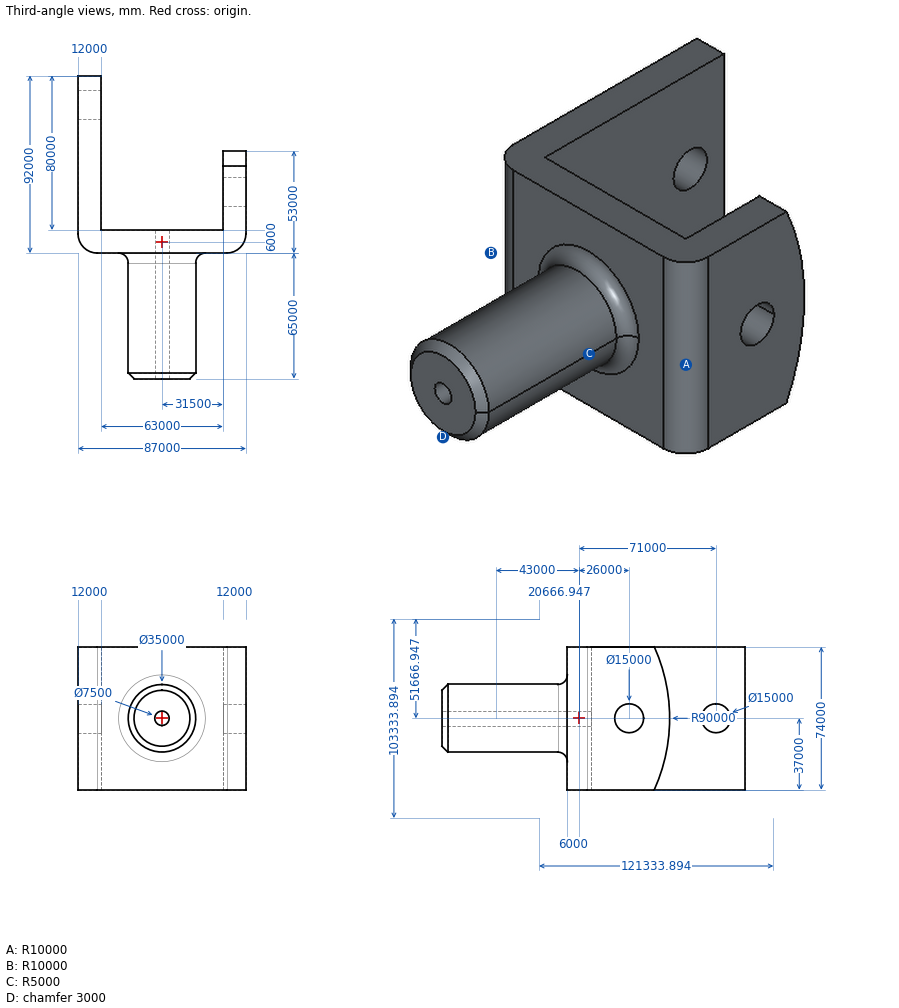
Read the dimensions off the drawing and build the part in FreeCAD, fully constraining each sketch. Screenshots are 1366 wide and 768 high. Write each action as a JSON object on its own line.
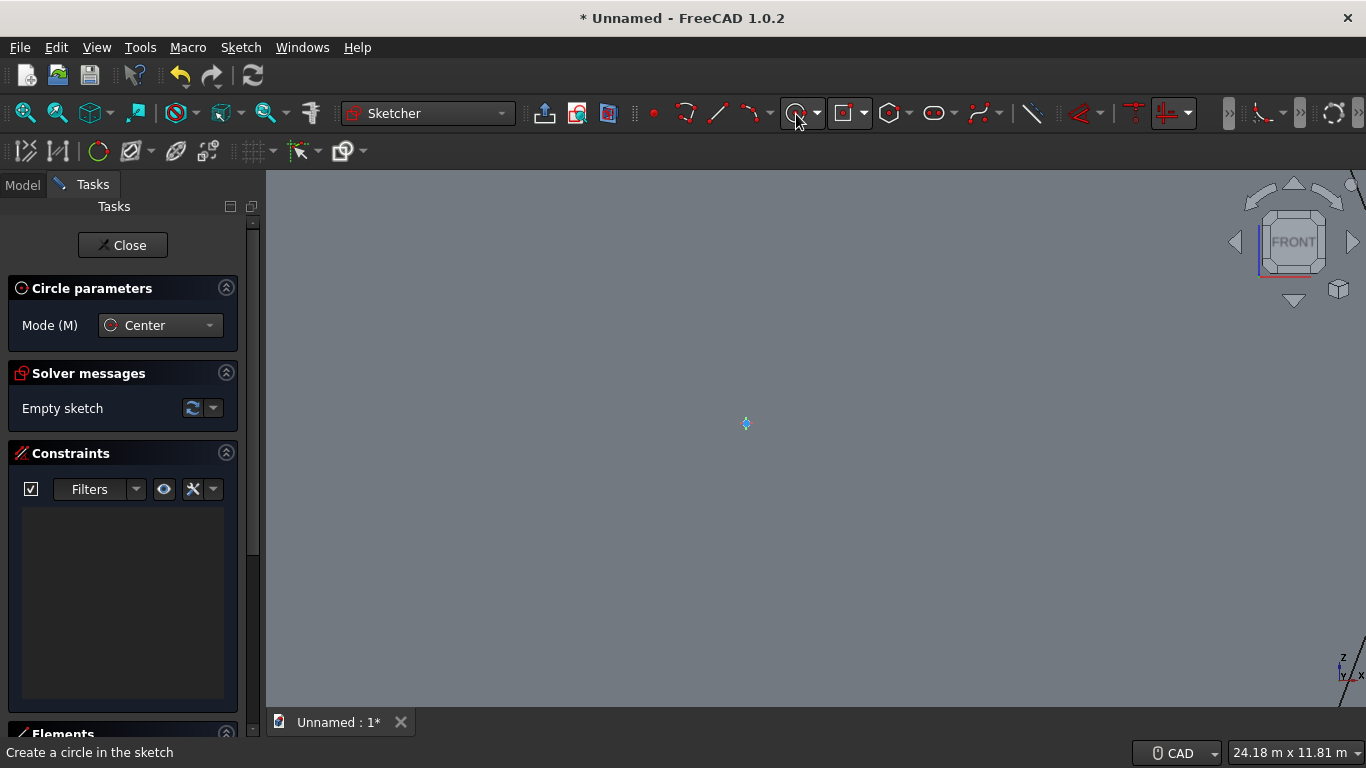
{"action": "left_click", "coordinate": [746, 423]}
{"action": "mouse_move", "coordinate": [867, 302]}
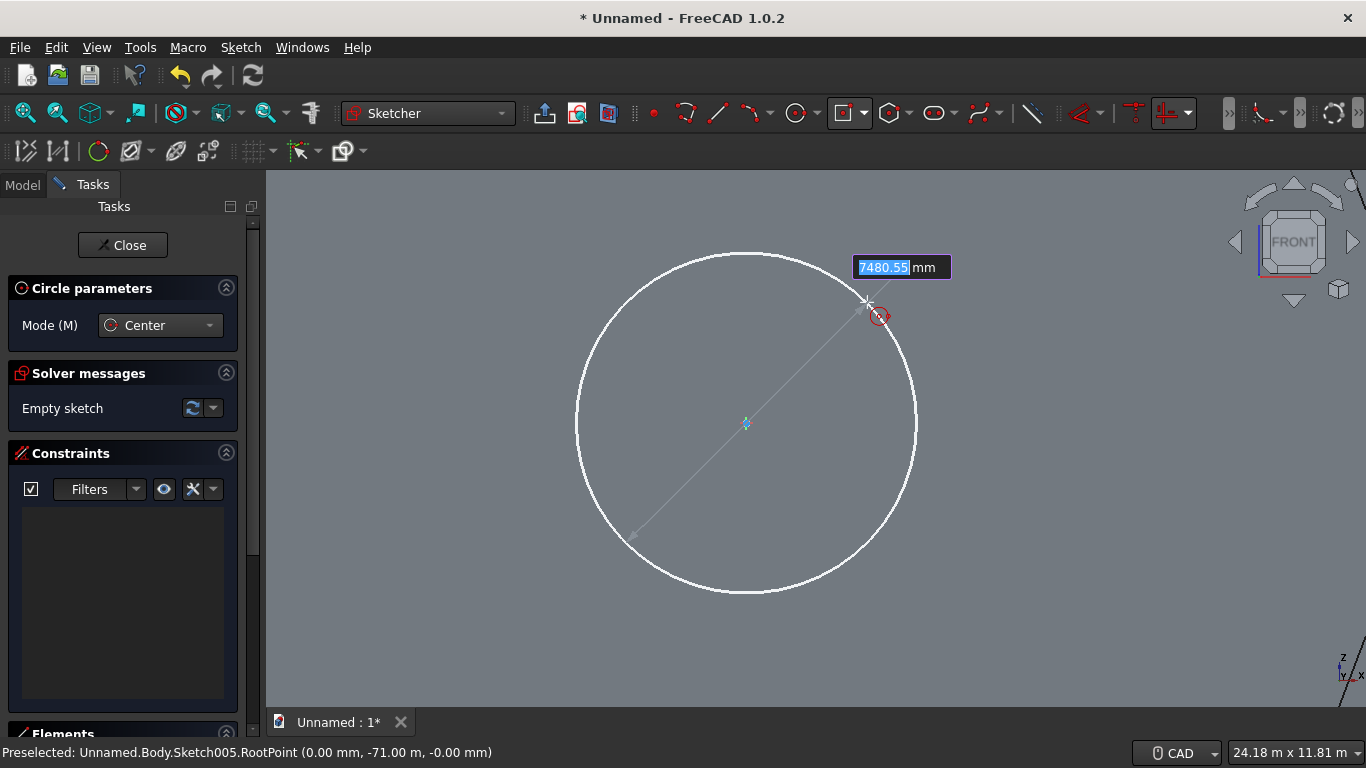
{"action": "type", "text": "7500"}
{"action": "key", "text": "Return"}
{"action": "key", "text": "Escape"}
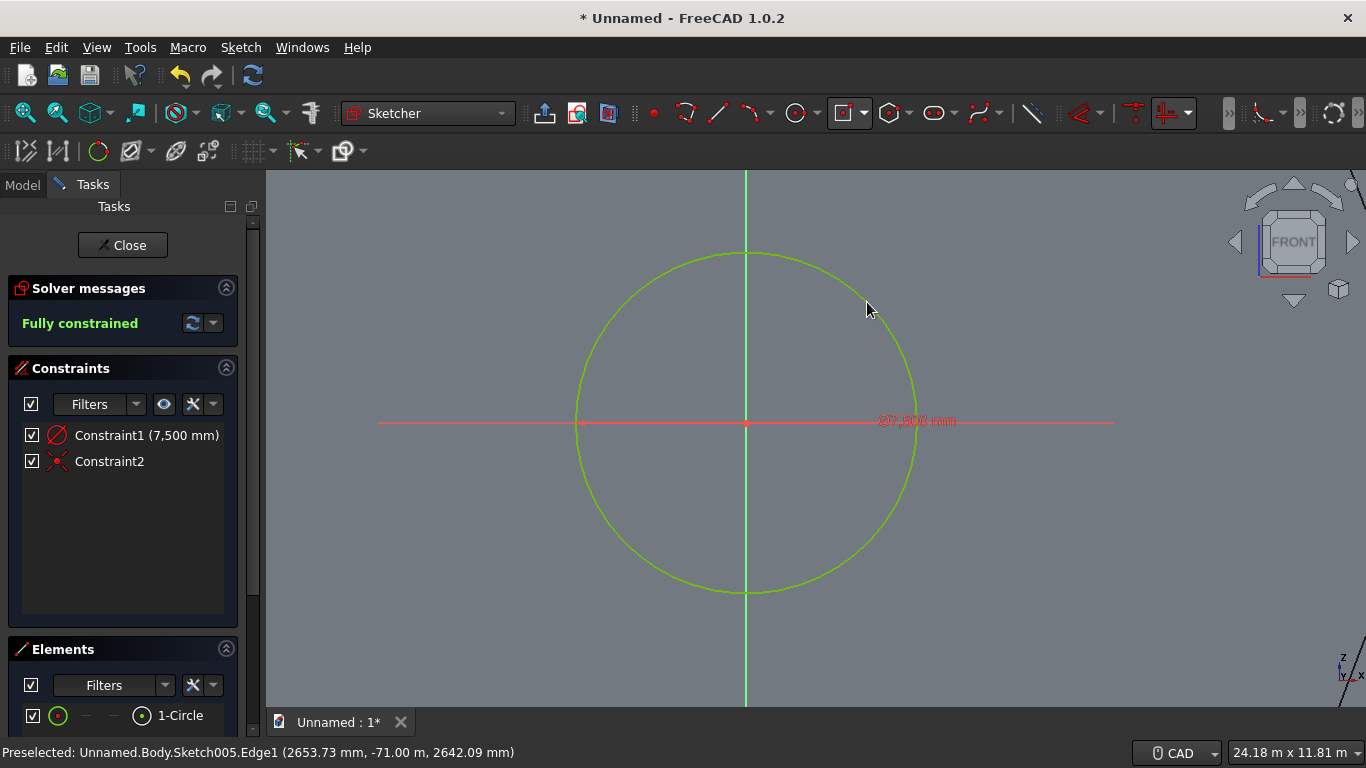
{"action": "left_click", "coordinate": [123, 245]}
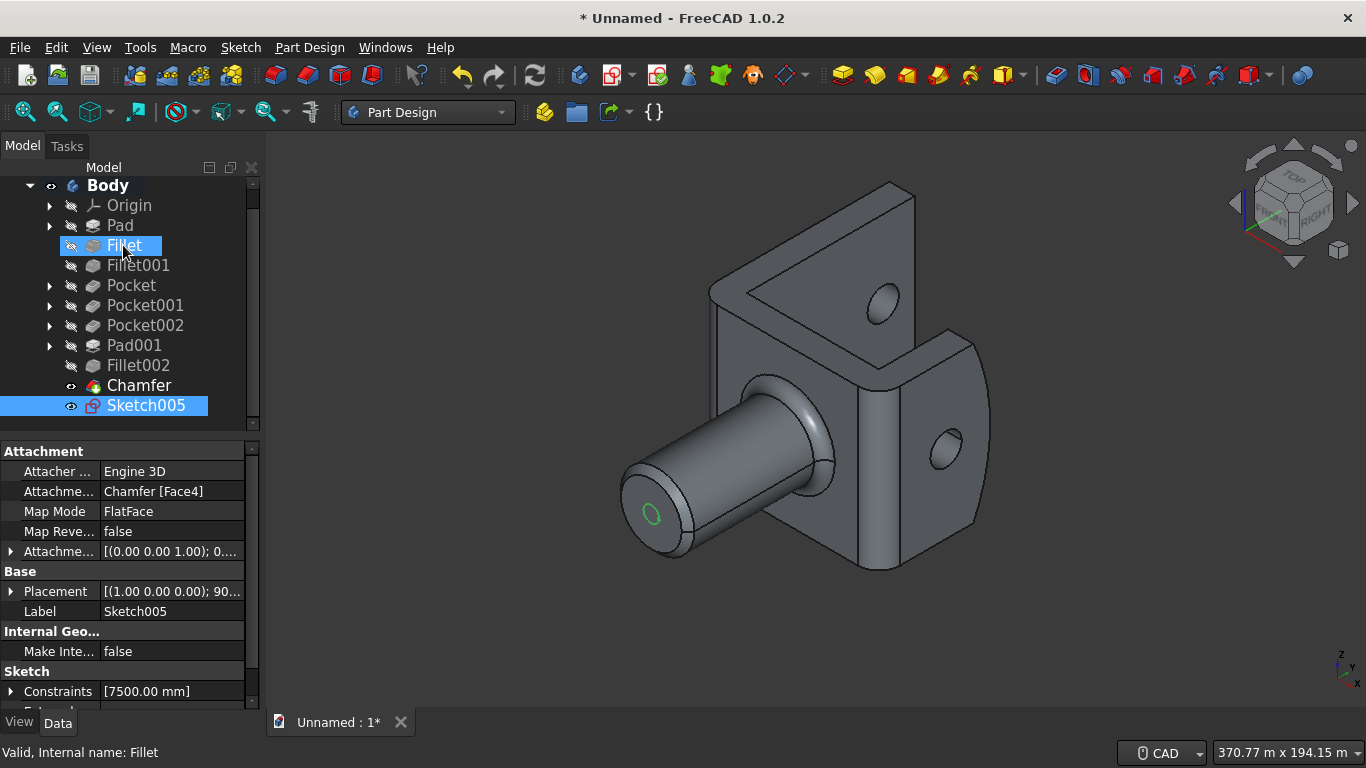
{"action": "left_click", "coordinate": [1058, 76]}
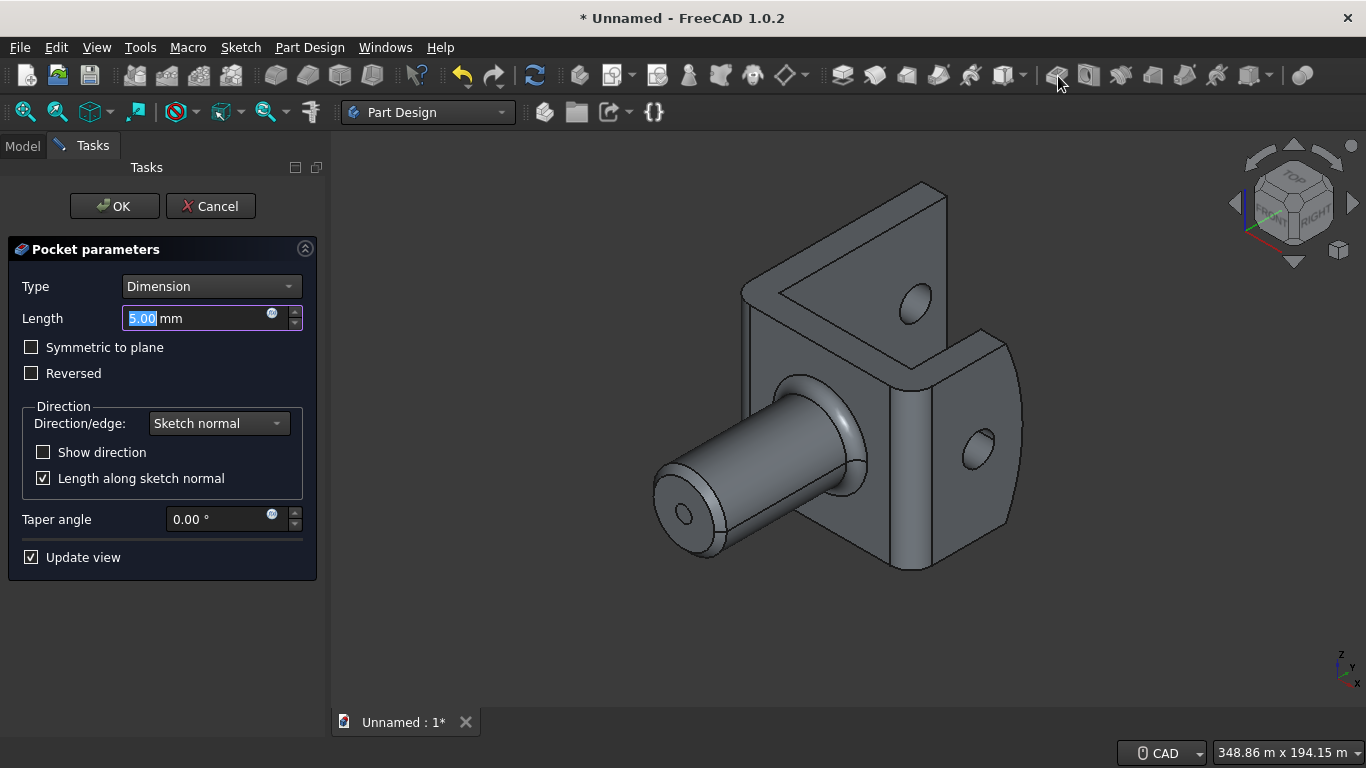
{"action": "left_click", "coordinate": [212, 286]}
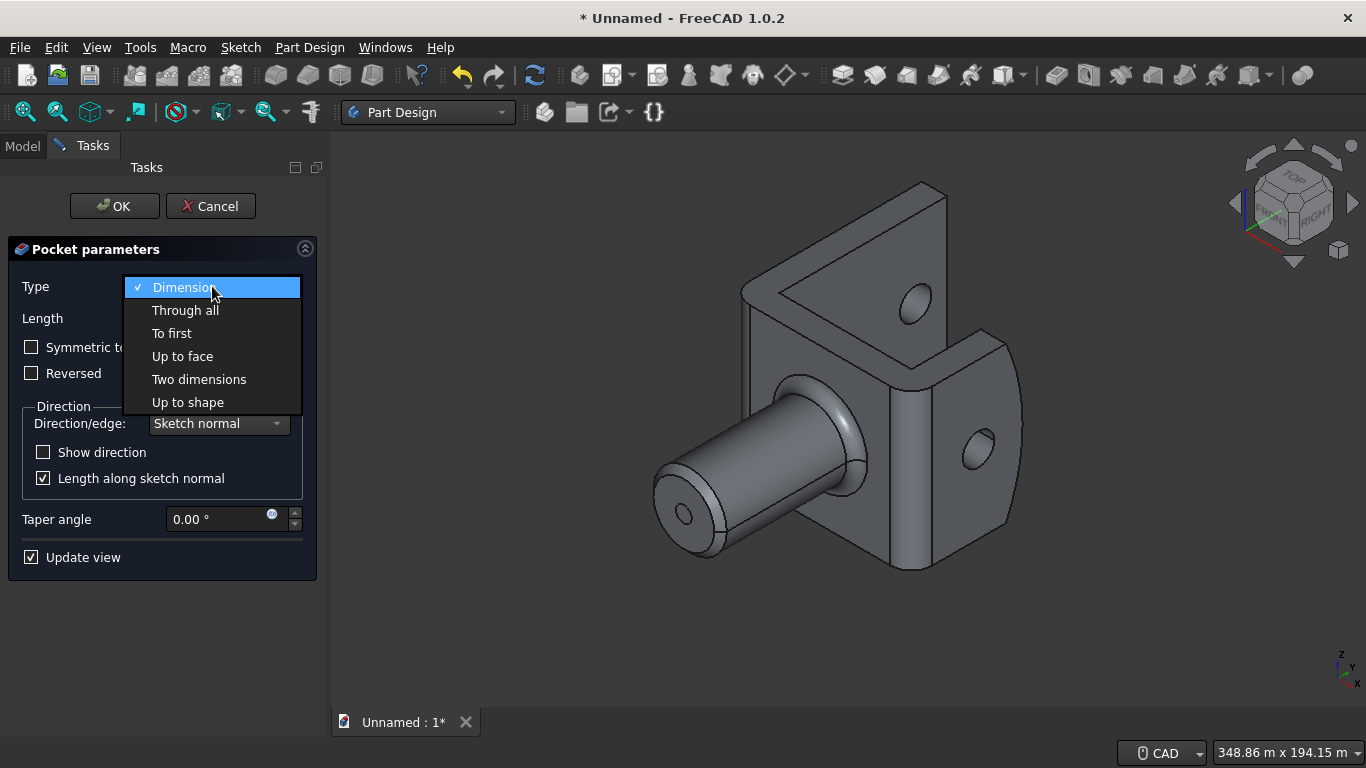
{"action": "left_click", "coordinate": [212, 310]}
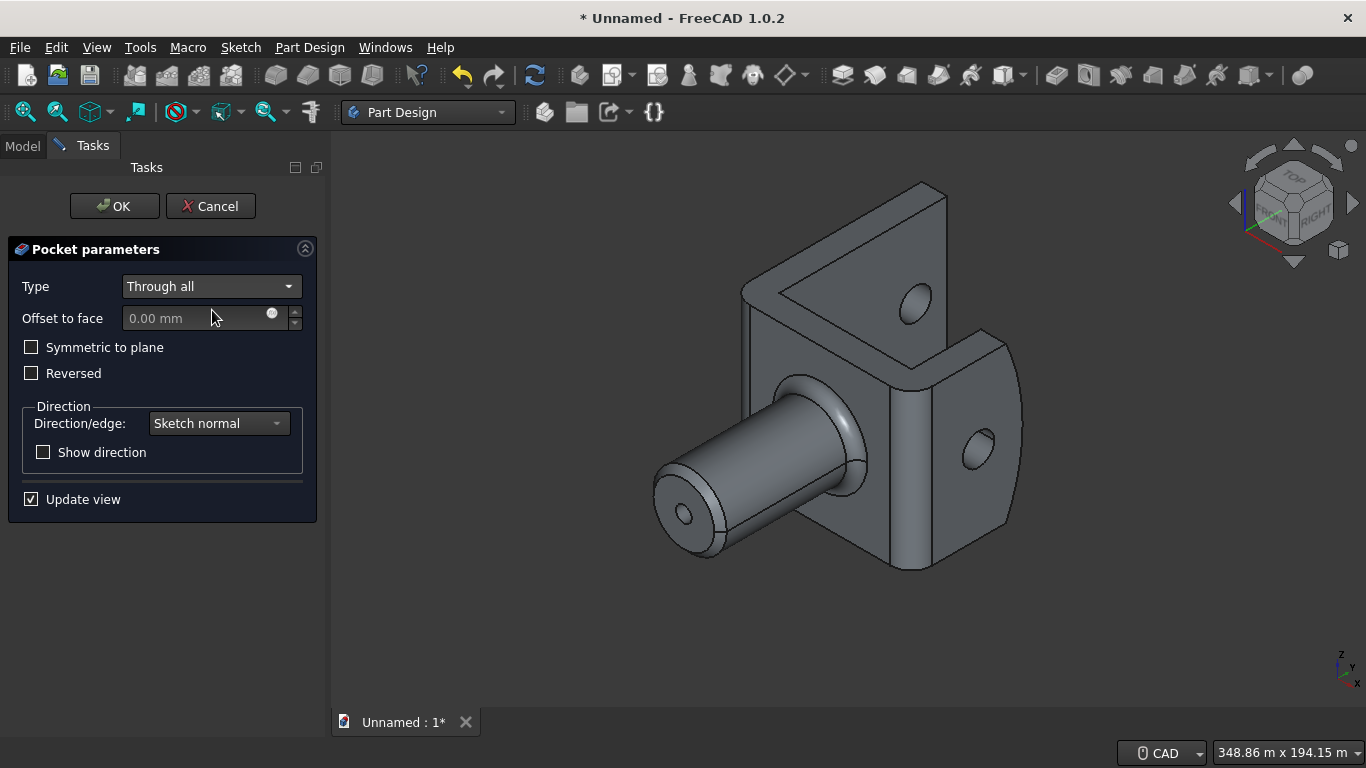
{"action": "left_click", "coordinate": [115, 206]}